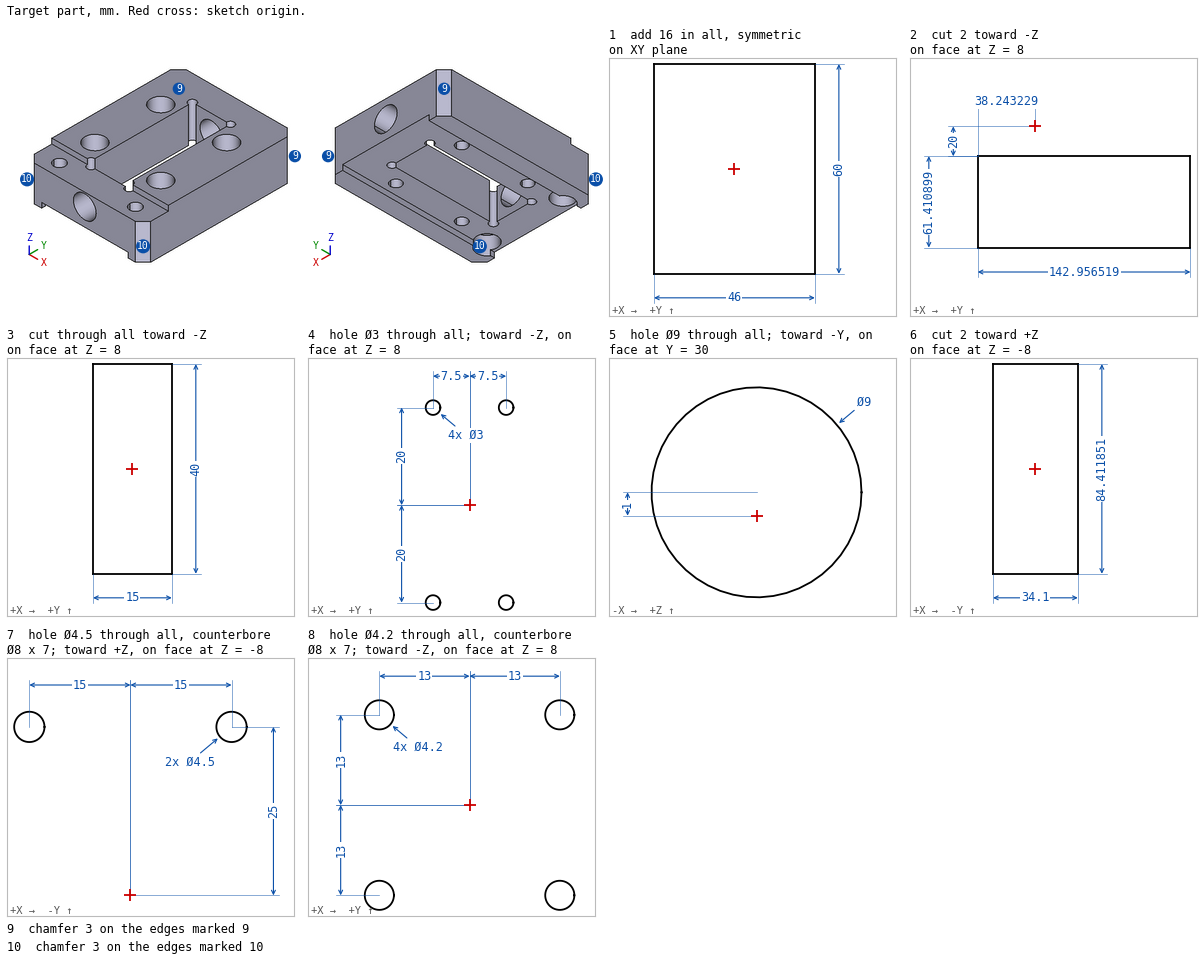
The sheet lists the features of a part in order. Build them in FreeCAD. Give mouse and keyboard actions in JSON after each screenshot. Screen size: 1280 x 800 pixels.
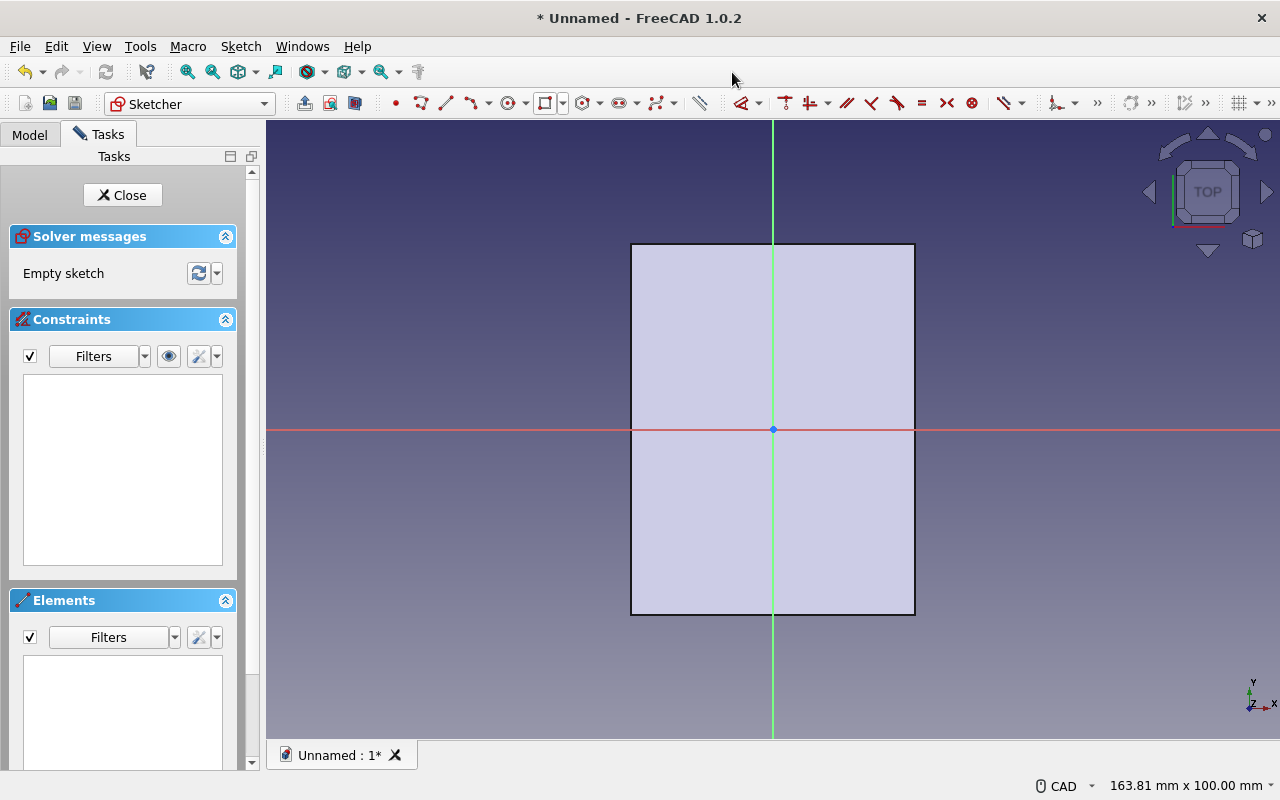
{"action": "scroll", "coordinate": [294, 148], "scroll_direction": "down", "scroll_amount": 2}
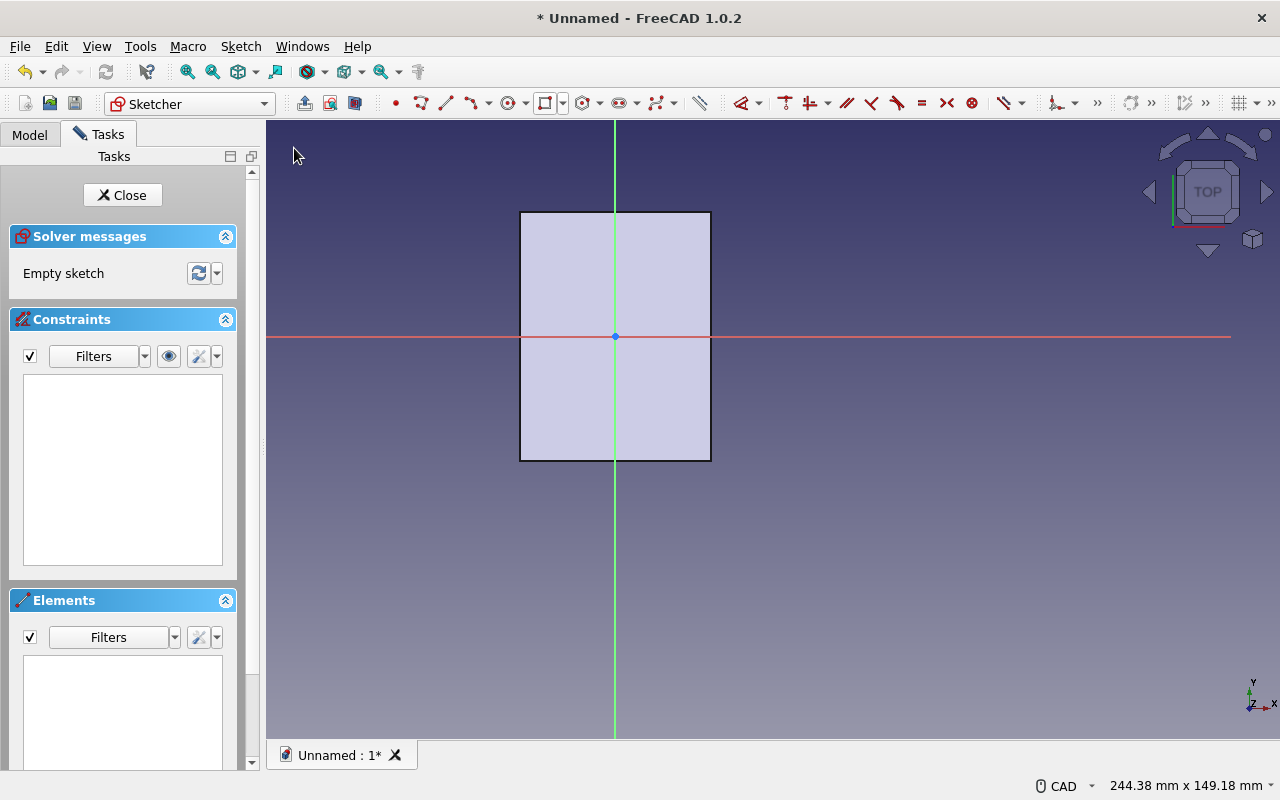
{"action": "left_click", "coordinate": [544, 104]}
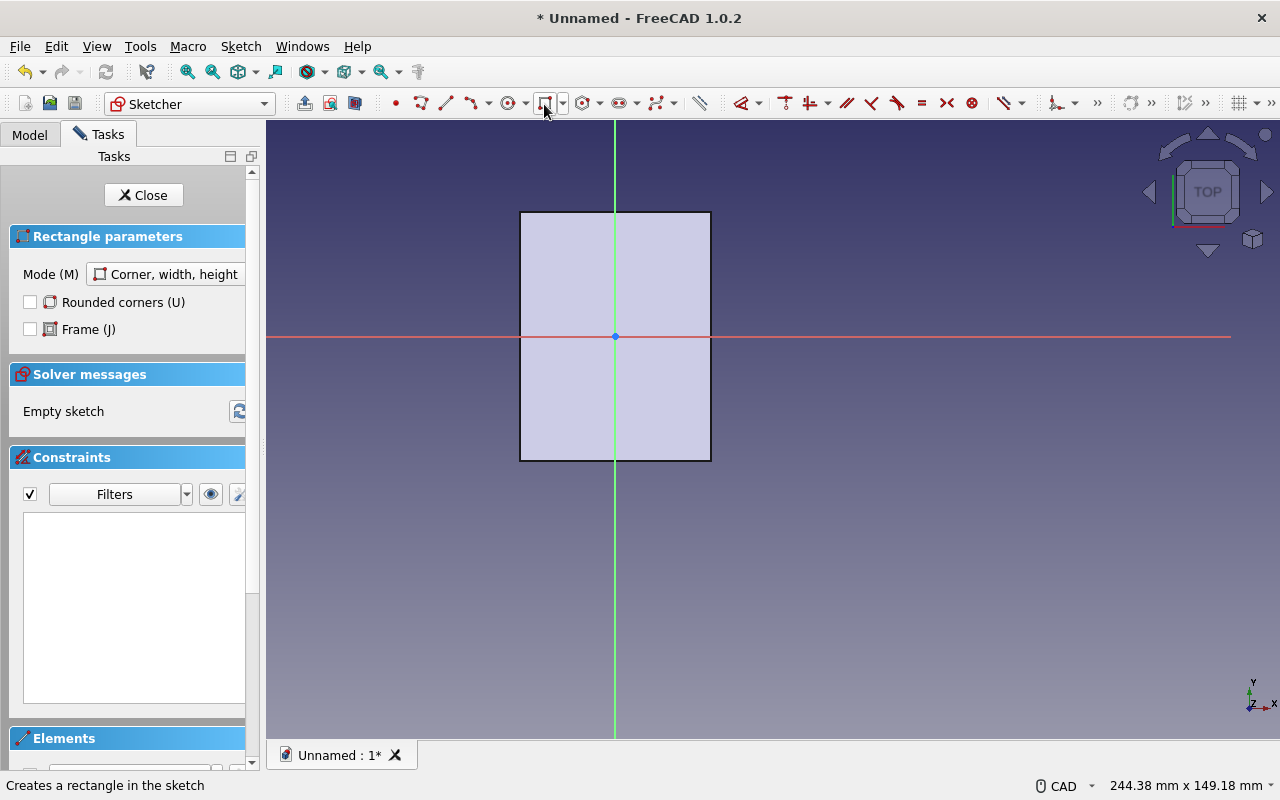
{"action": "left_click", "coordinate": [456, 420]}
{"action": "left_click", "coordinate": [1050, 675]}
{"action": "key", "text": "Escape"}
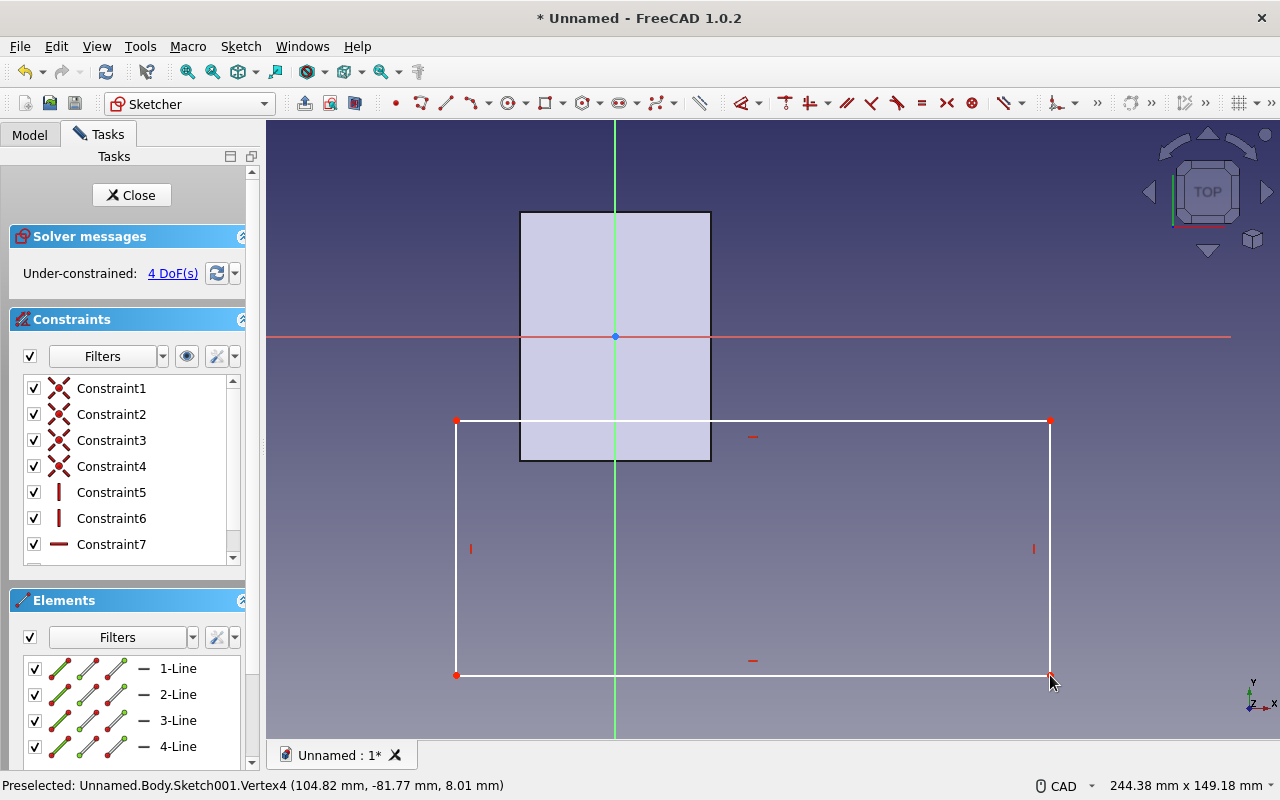
{"action": "left_click", "coordinate": [740, 104]}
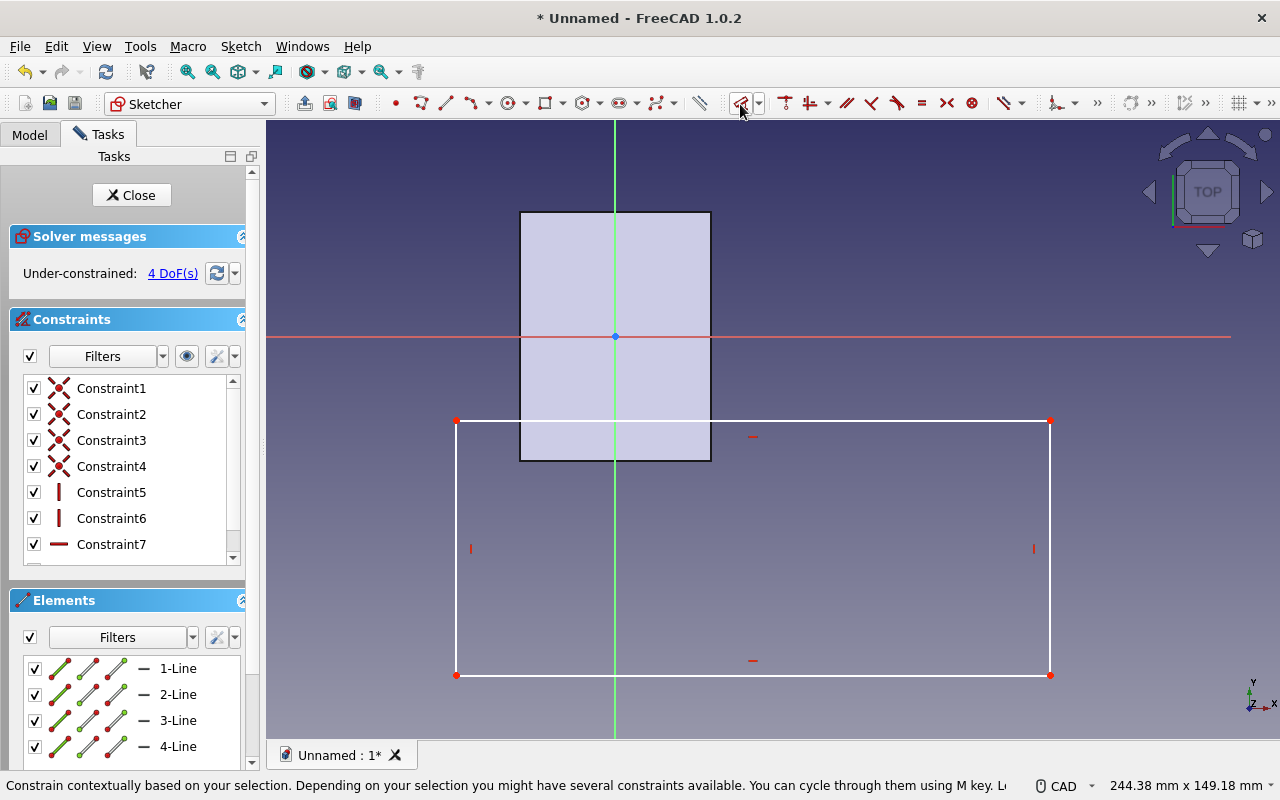
{"action": "left_click", "coordinate": [456, 421]}
{"action": "left_click", "coordinate": [422, 379]}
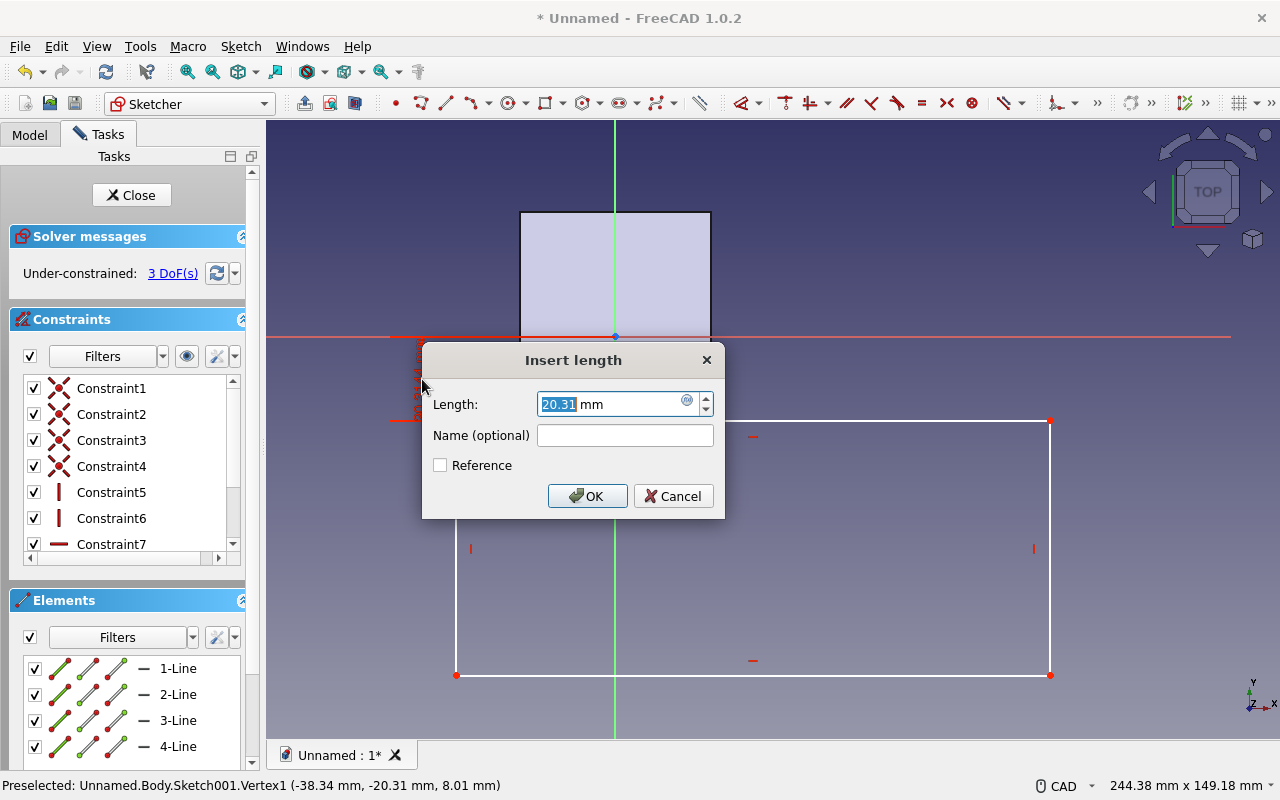
{"action": "type", "text": "20"}
{"action": "key", "text": "Return"}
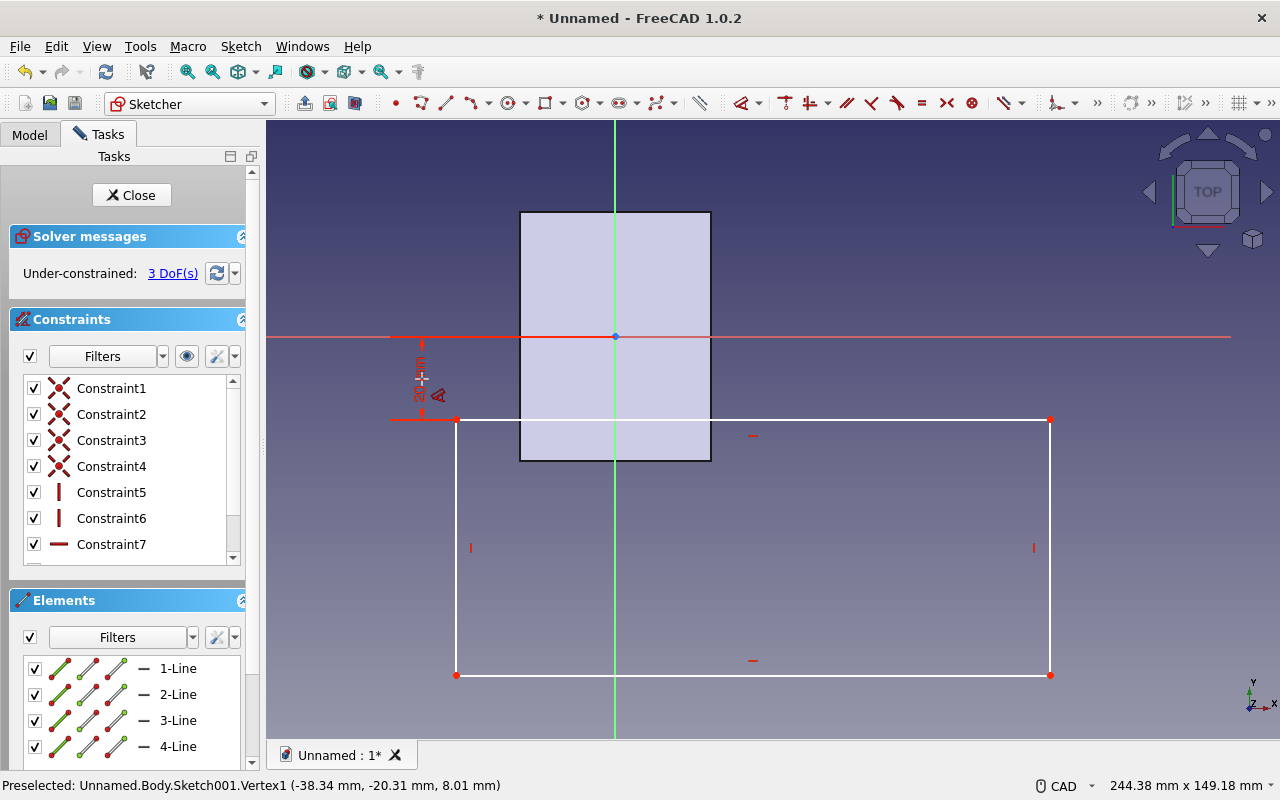
{"action": "left_click", "coordinate": [456, 497]}
{"action": "left_click", "coordinate": [422, 548]}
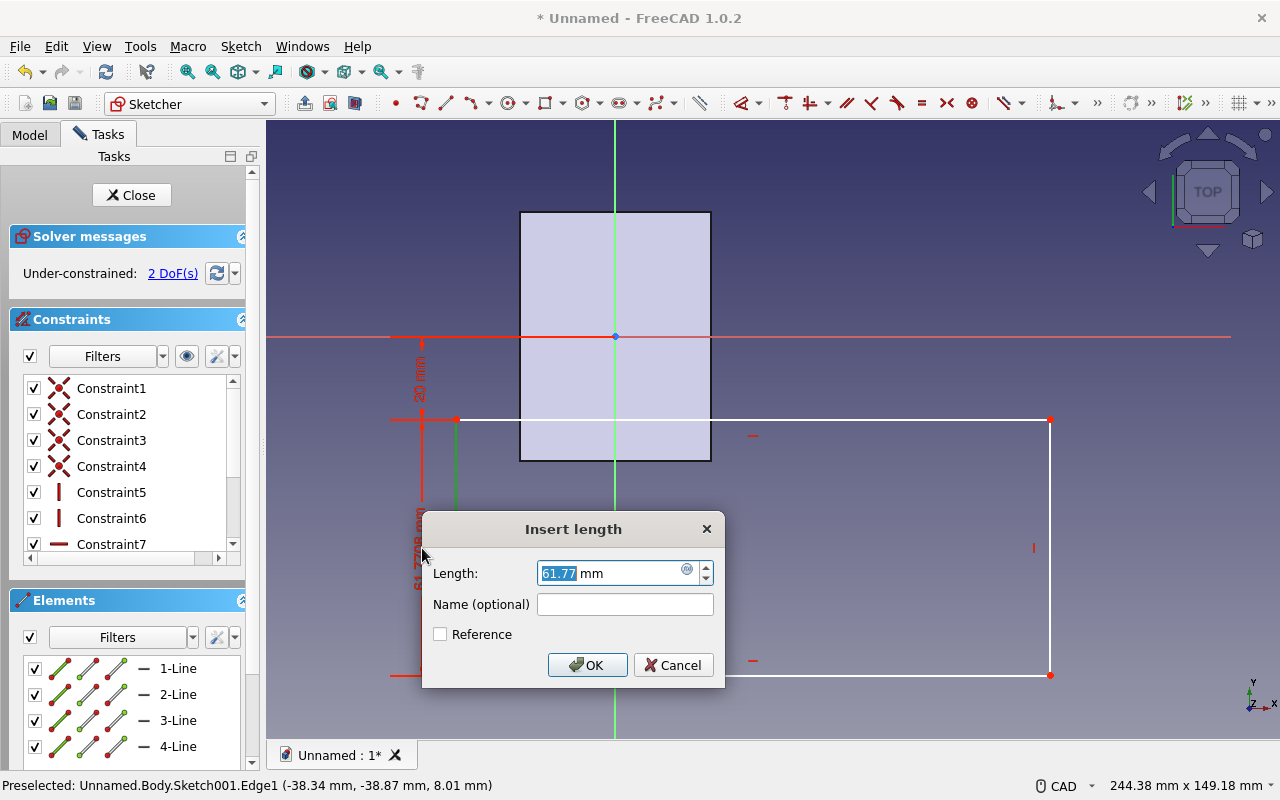
{"action": "type", "text": "61.410899"}
{"action": "key", "text": "Return"}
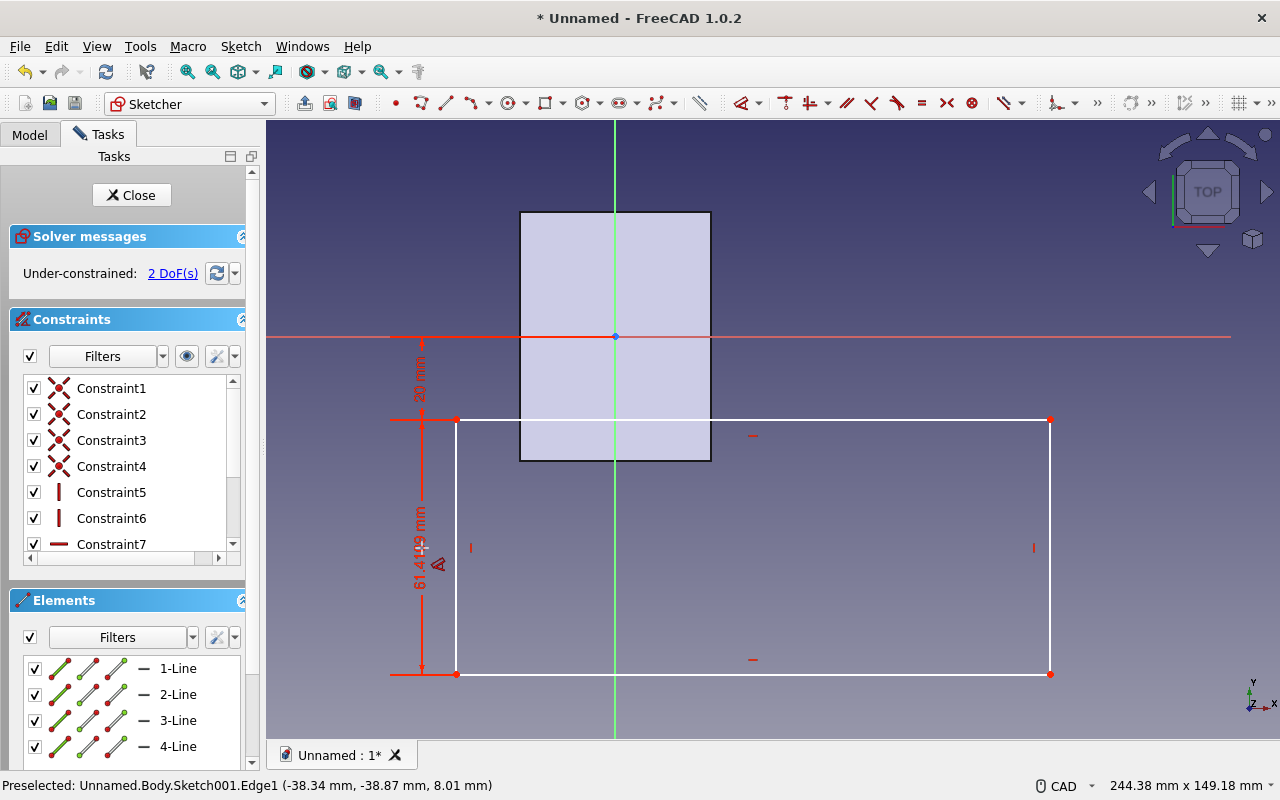
{"action": "left_click", "coordinate": [634, 675]}
{"action": "left_click", "coordinate": [753, 709]}